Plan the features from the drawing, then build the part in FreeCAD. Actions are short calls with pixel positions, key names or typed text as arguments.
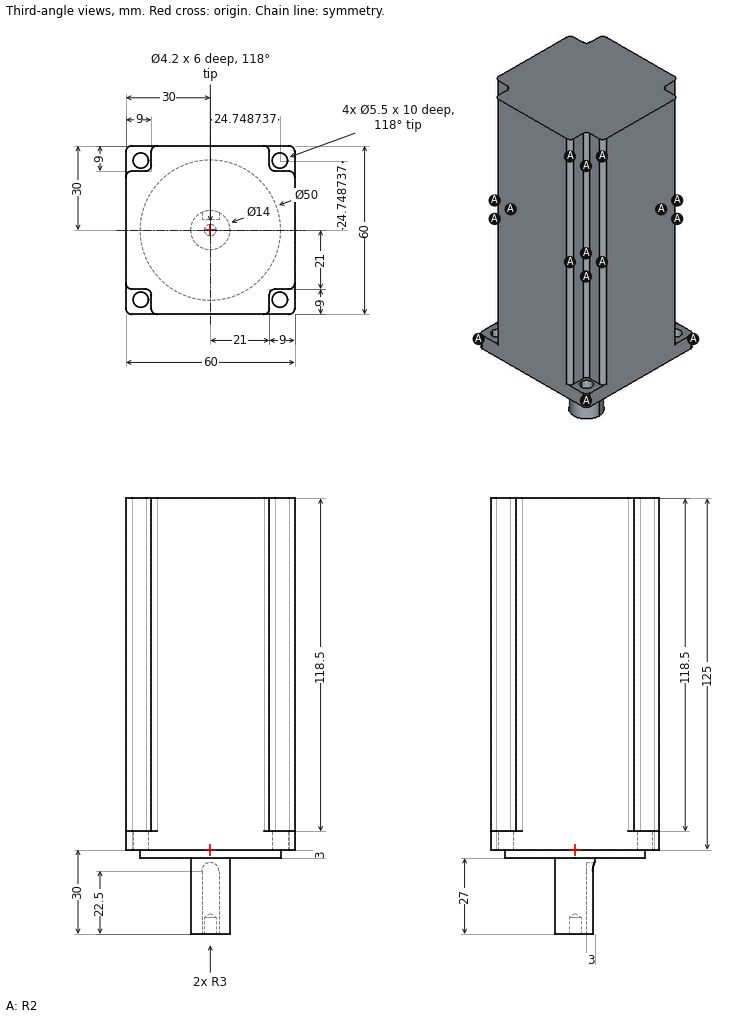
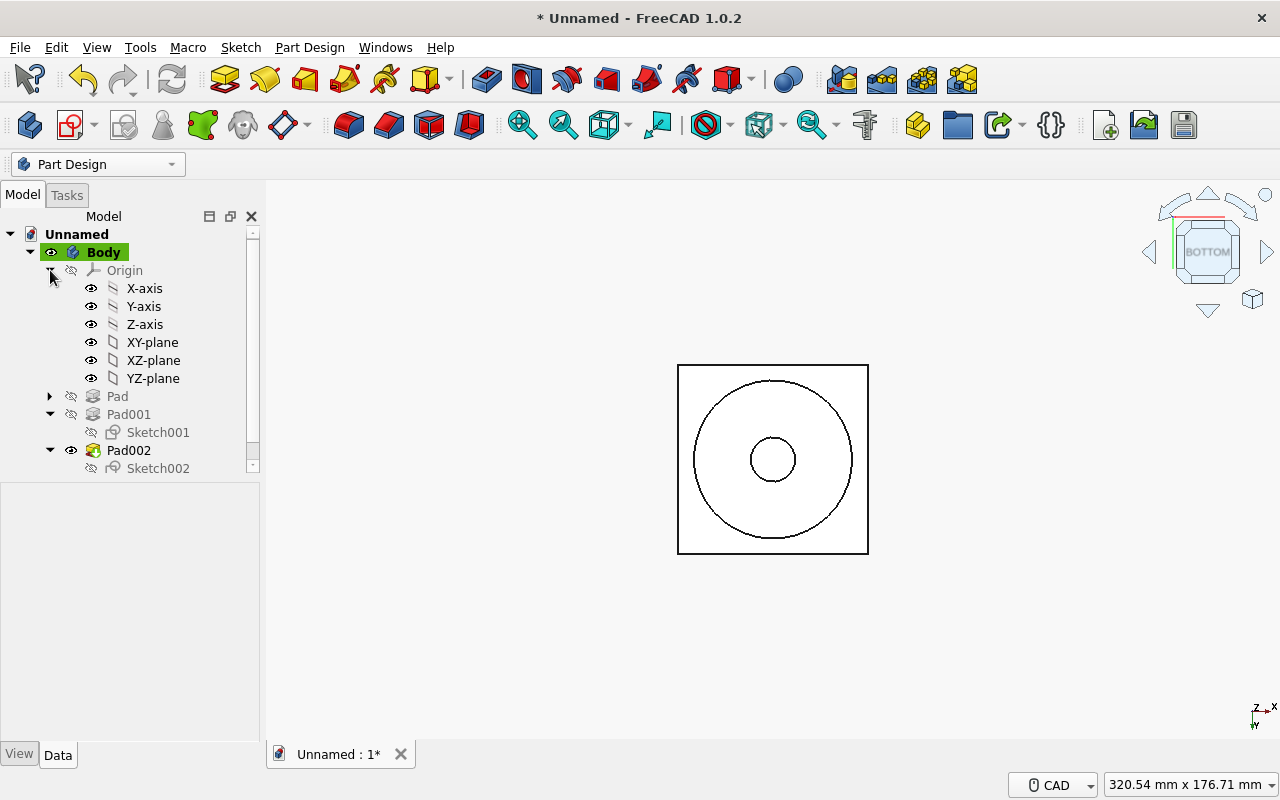
click(136, 360)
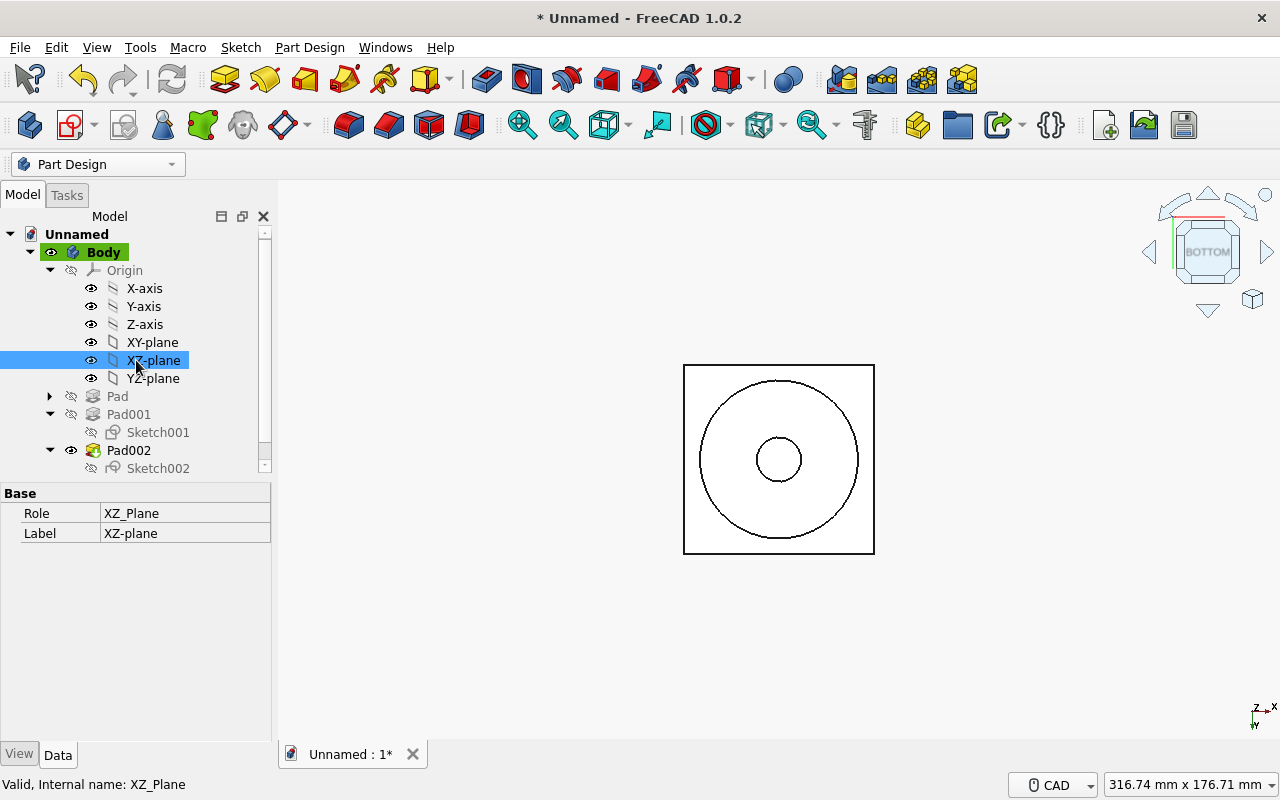
click(284, 126)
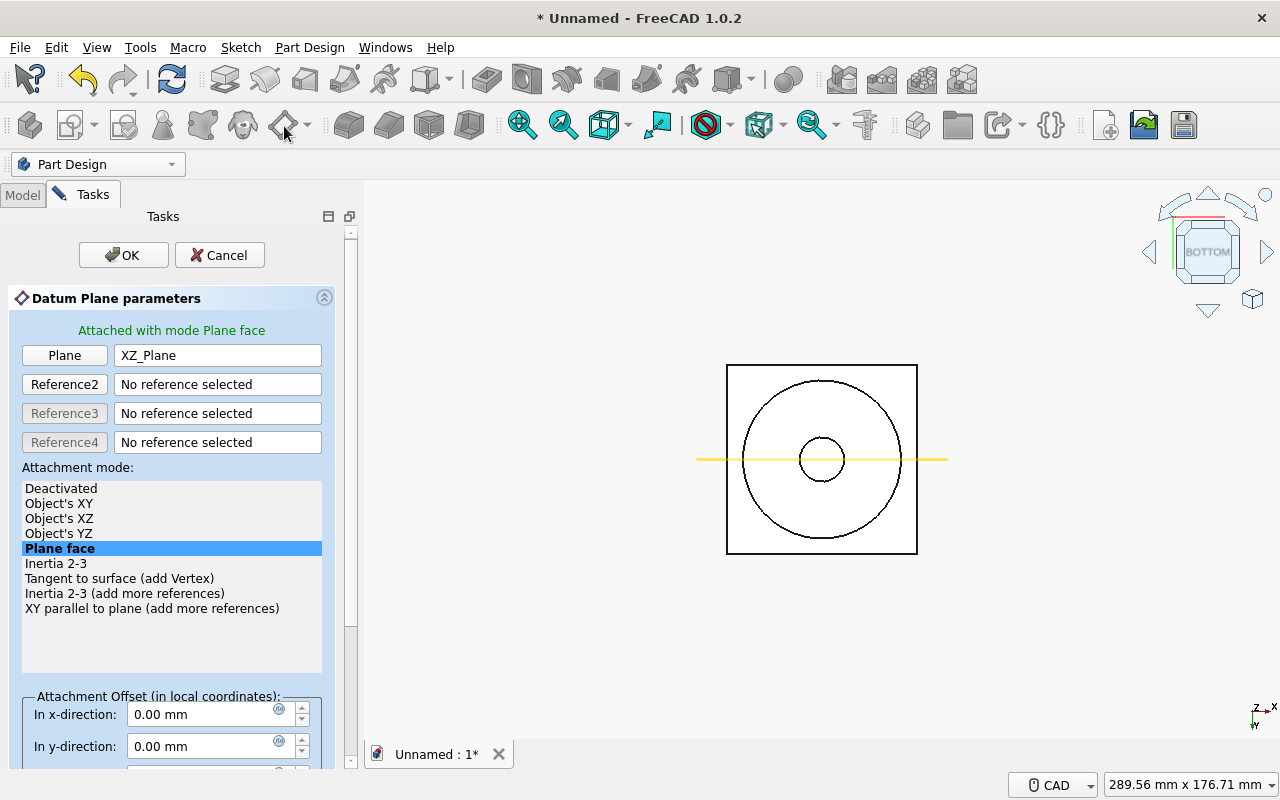
scroll(351, 497, down, 2)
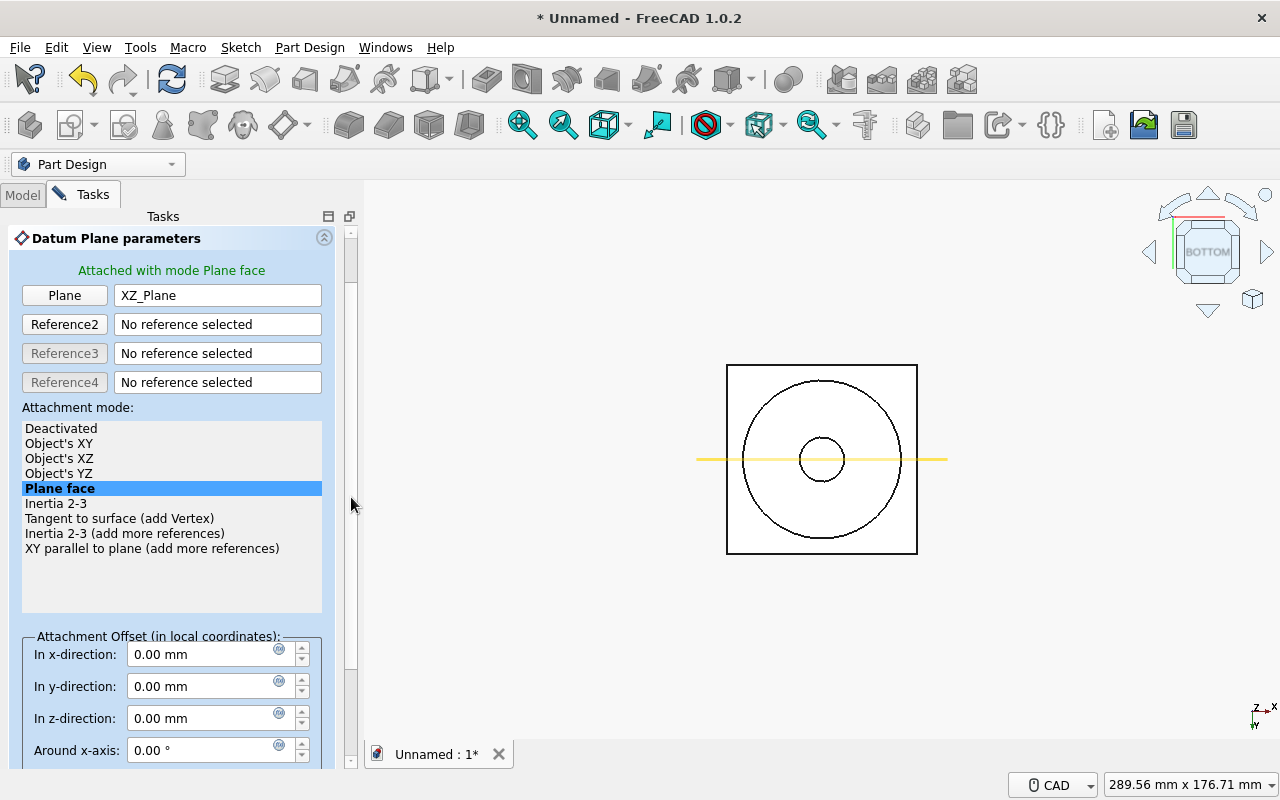
triple_click(210, 658)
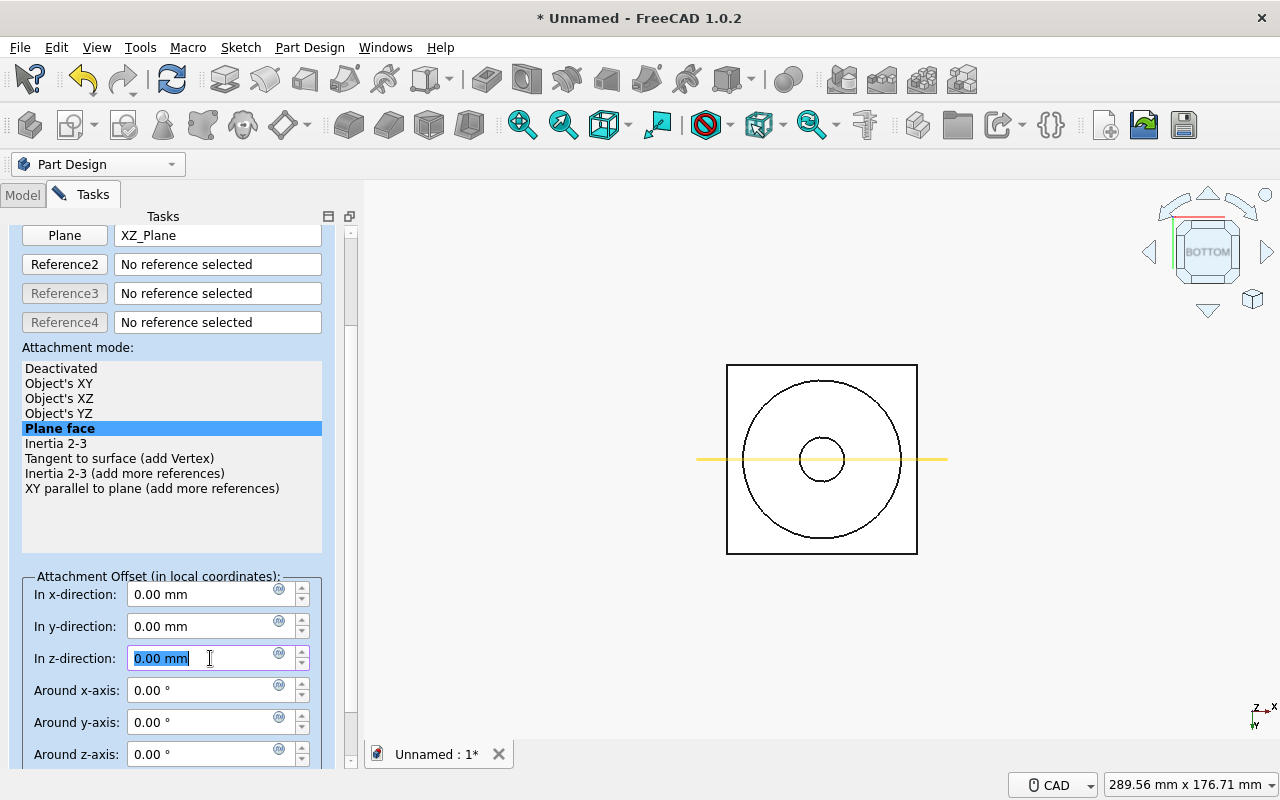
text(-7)
key(Tab)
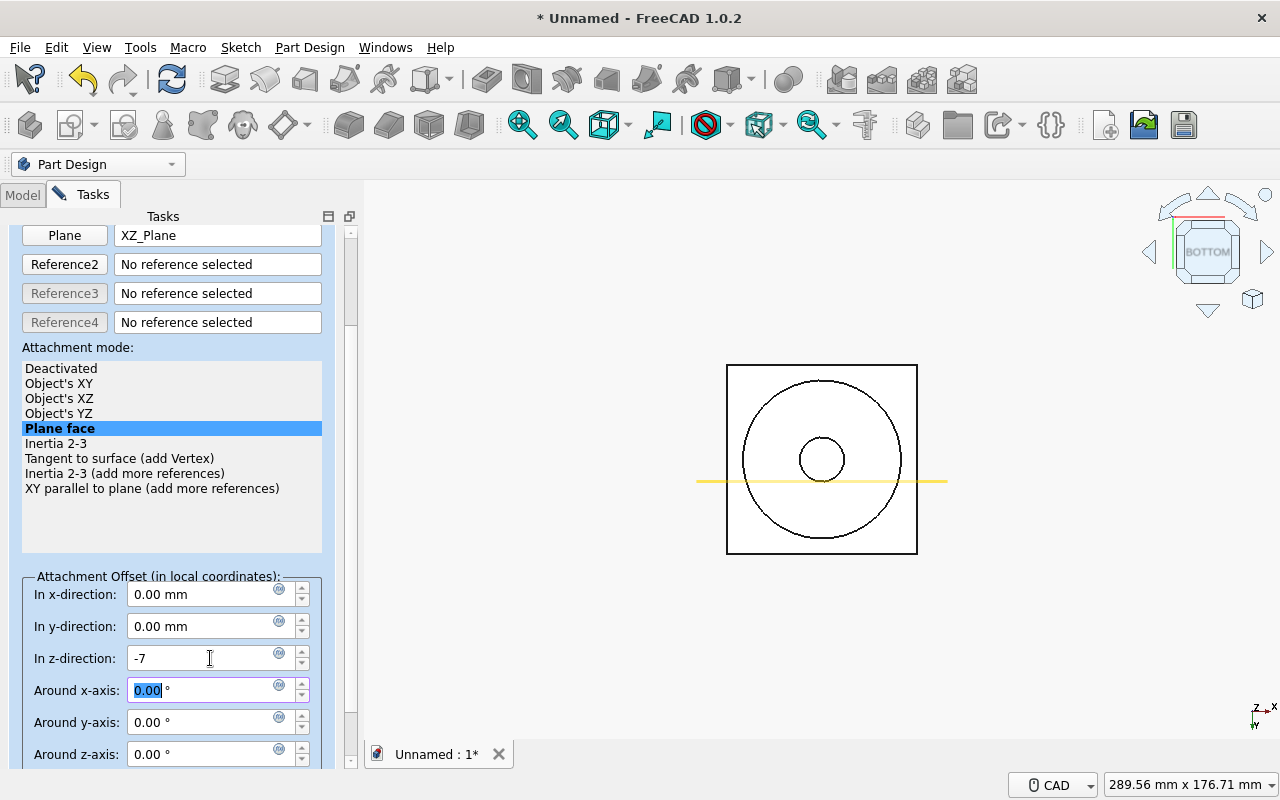
scroll(351, 497, up, 3)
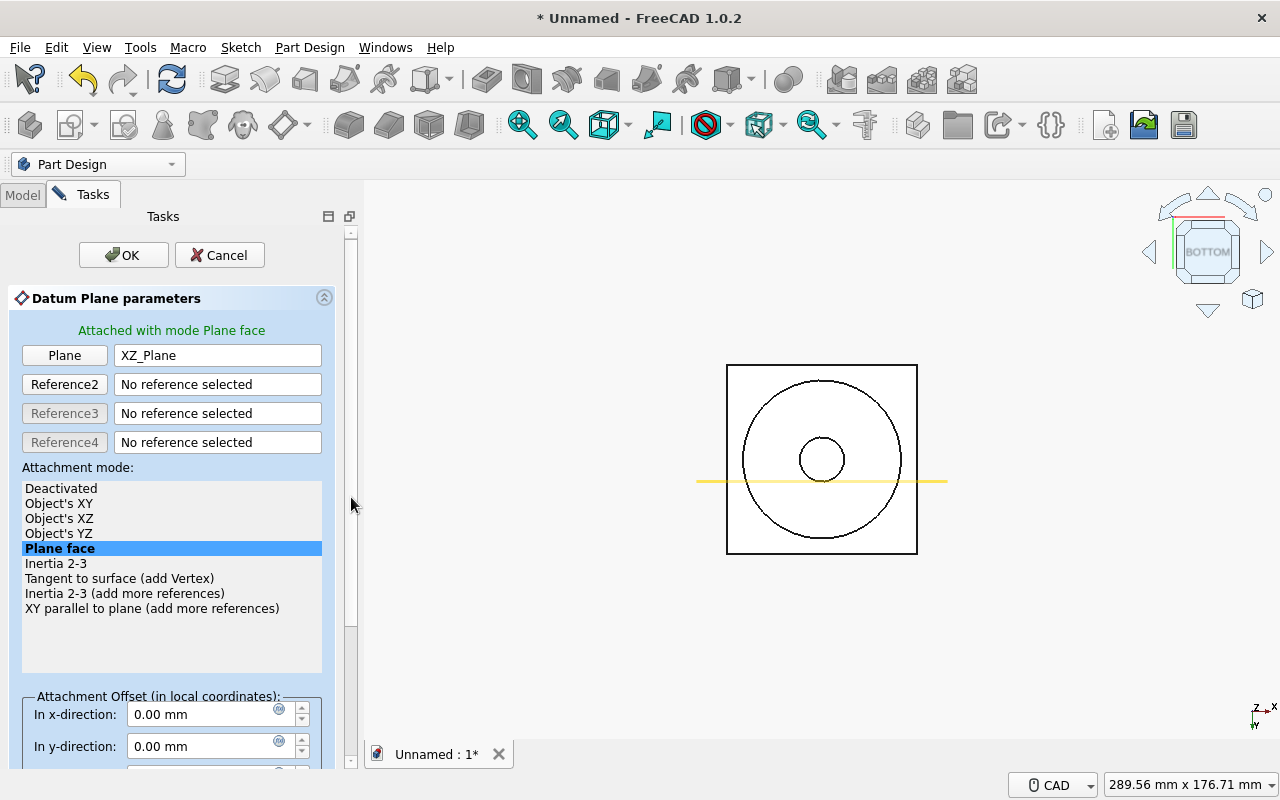
click(124, 255)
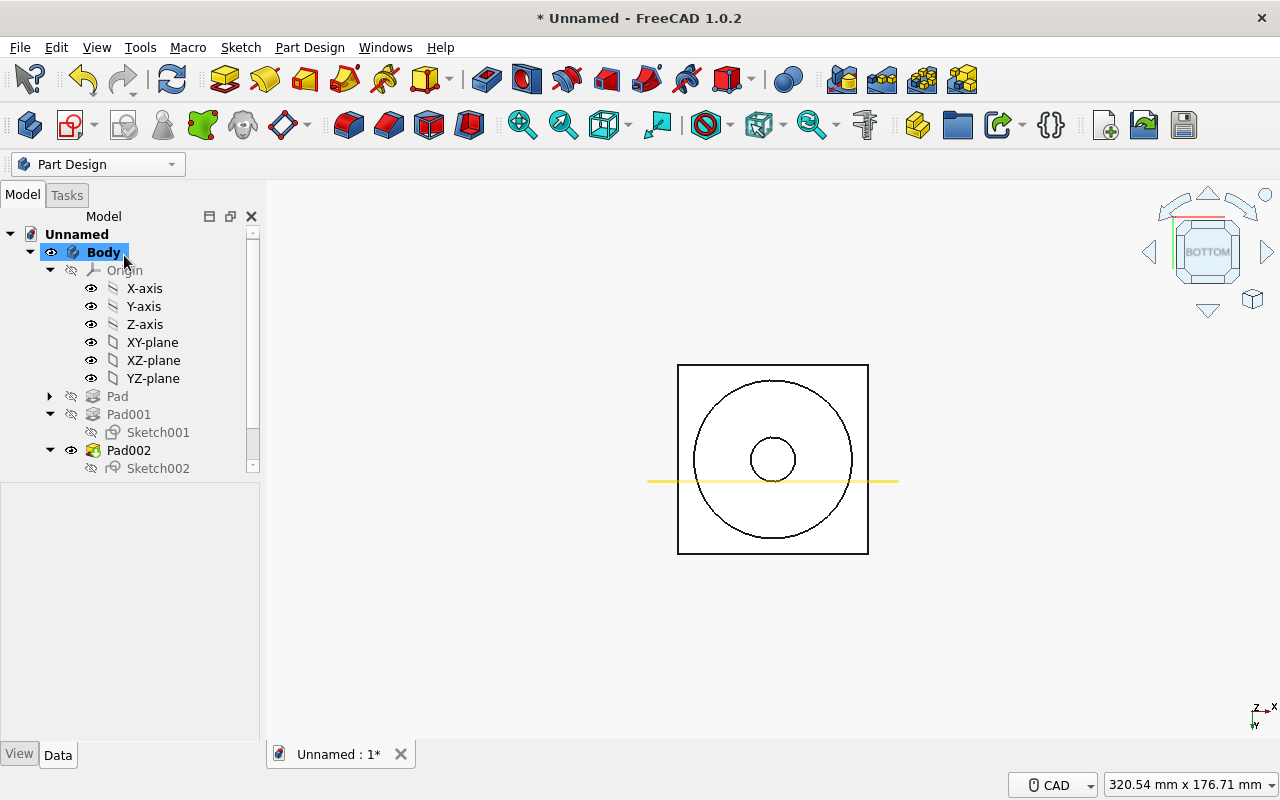
scroll(100, 356, down, 3)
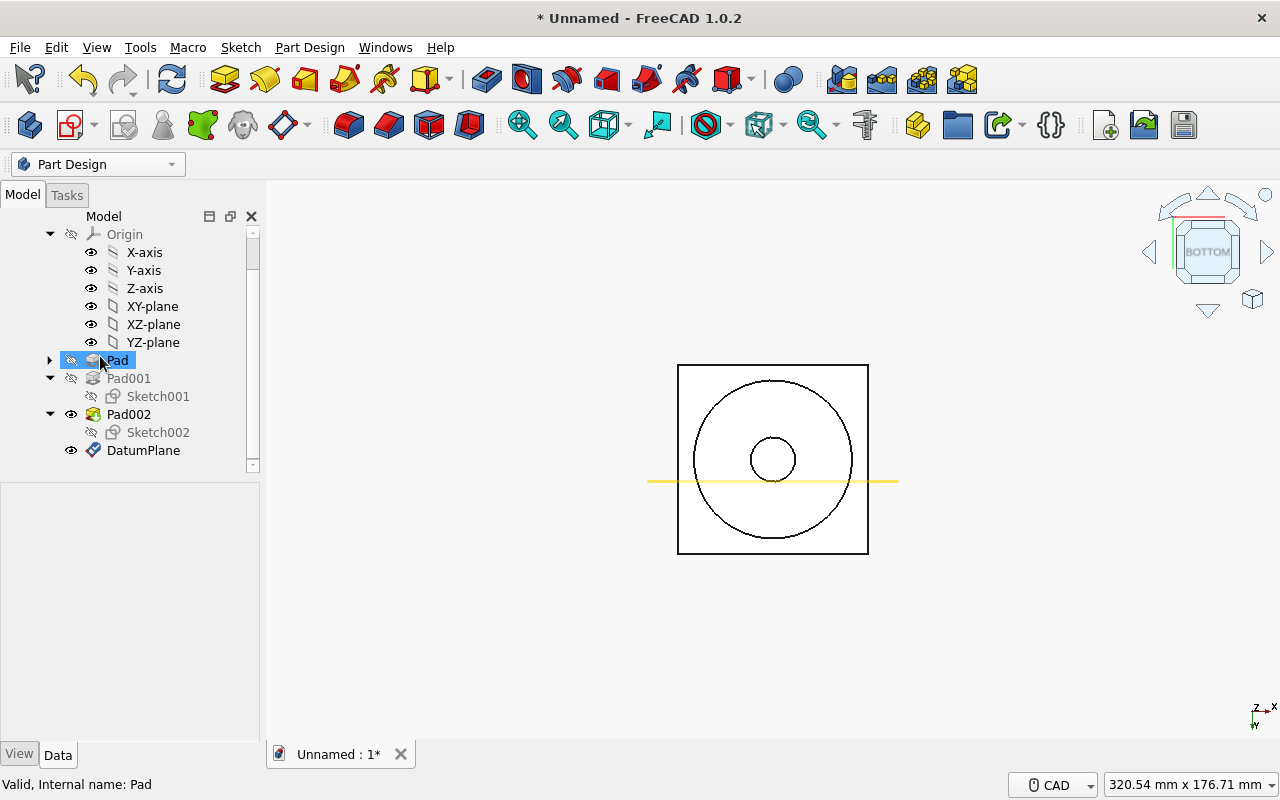
click(116, 450)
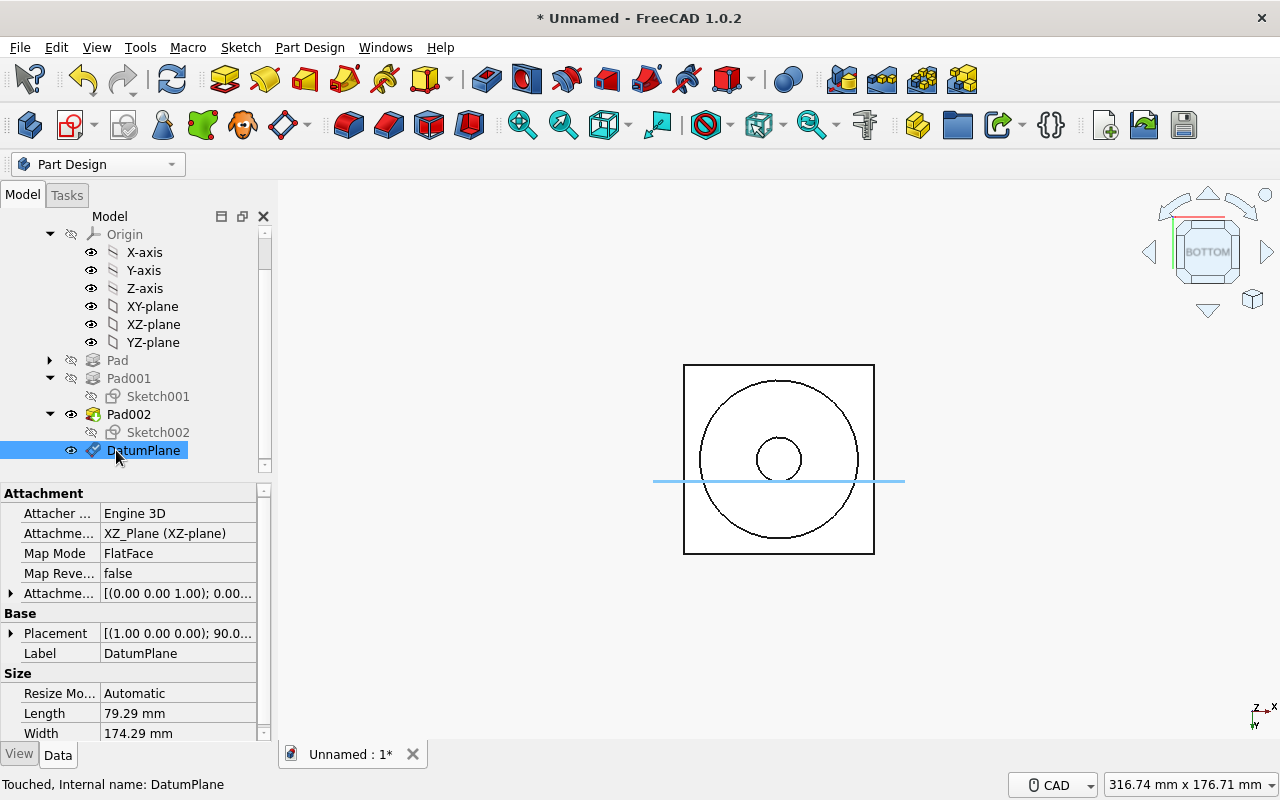
click(70, 126)